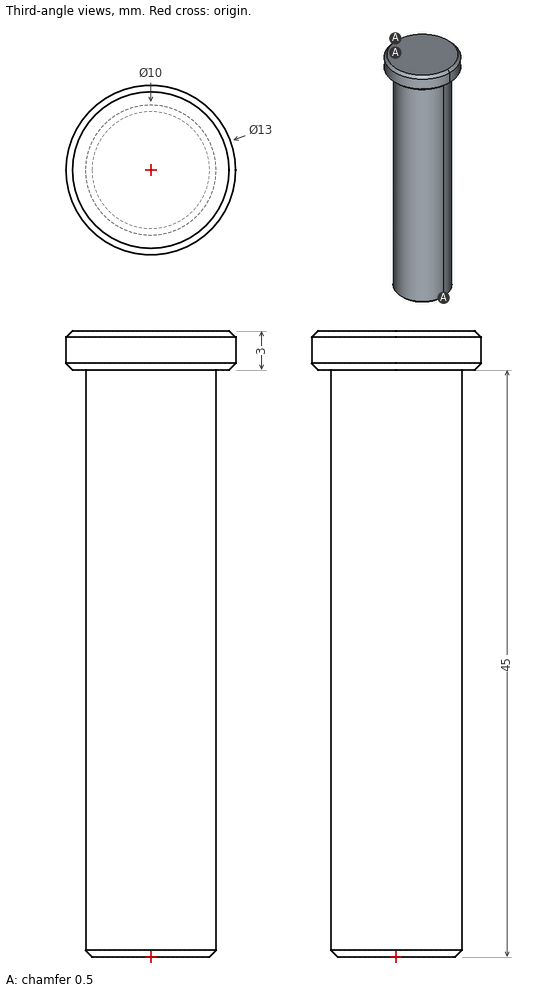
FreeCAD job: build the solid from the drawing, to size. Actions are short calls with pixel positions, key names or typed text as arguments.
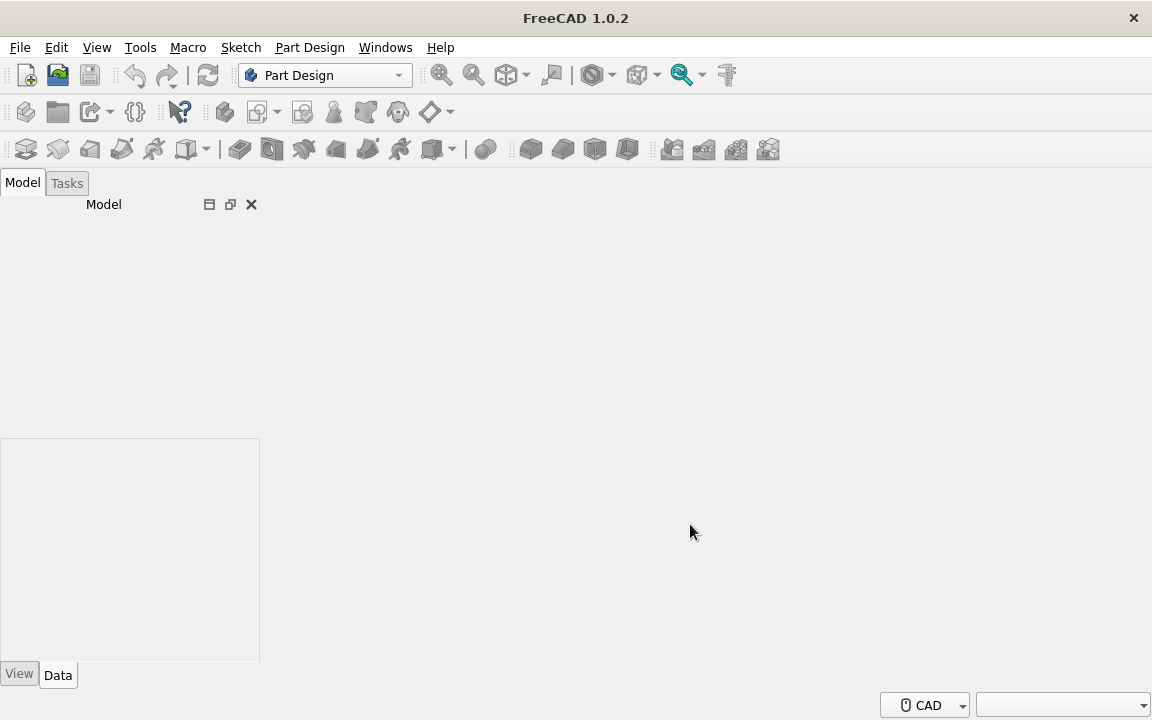
key(ctrl+n)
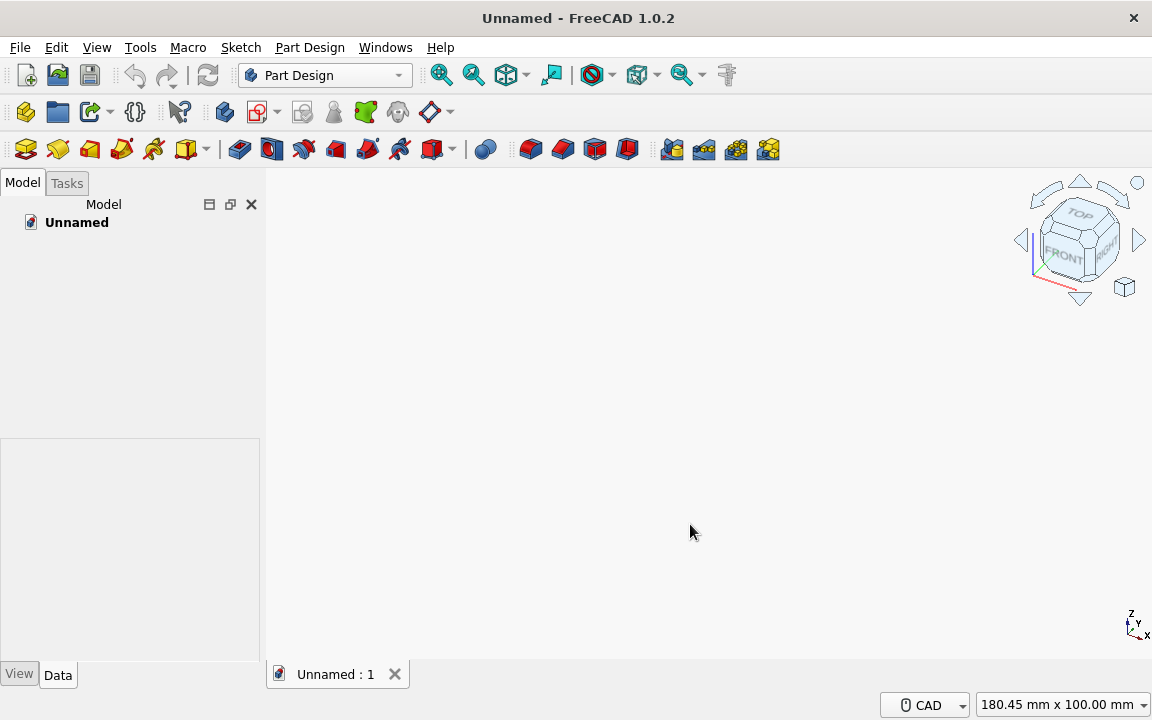
click(258, 112)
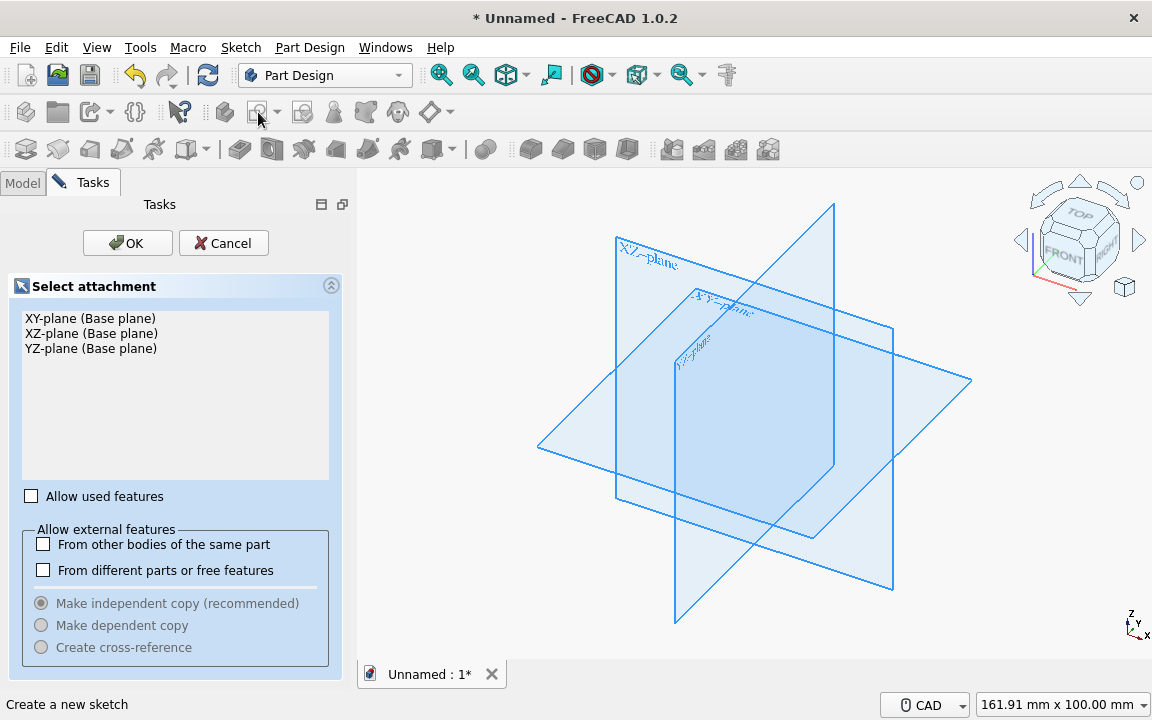
click(82, 318)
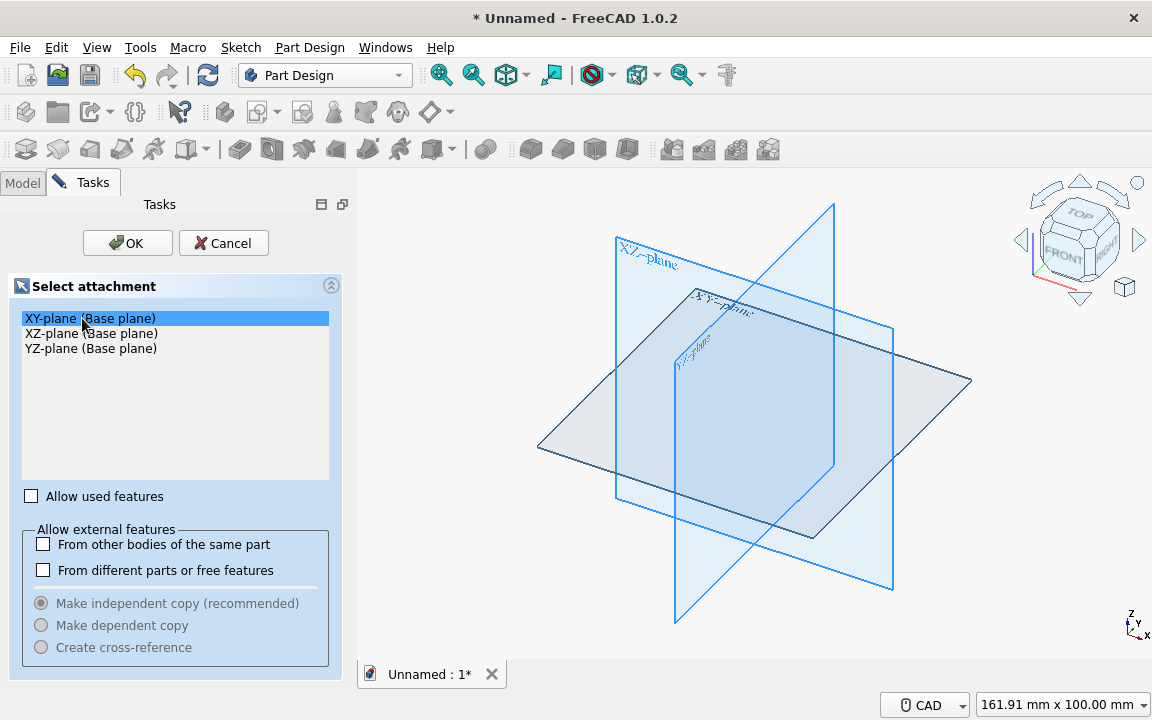
click(128, 243)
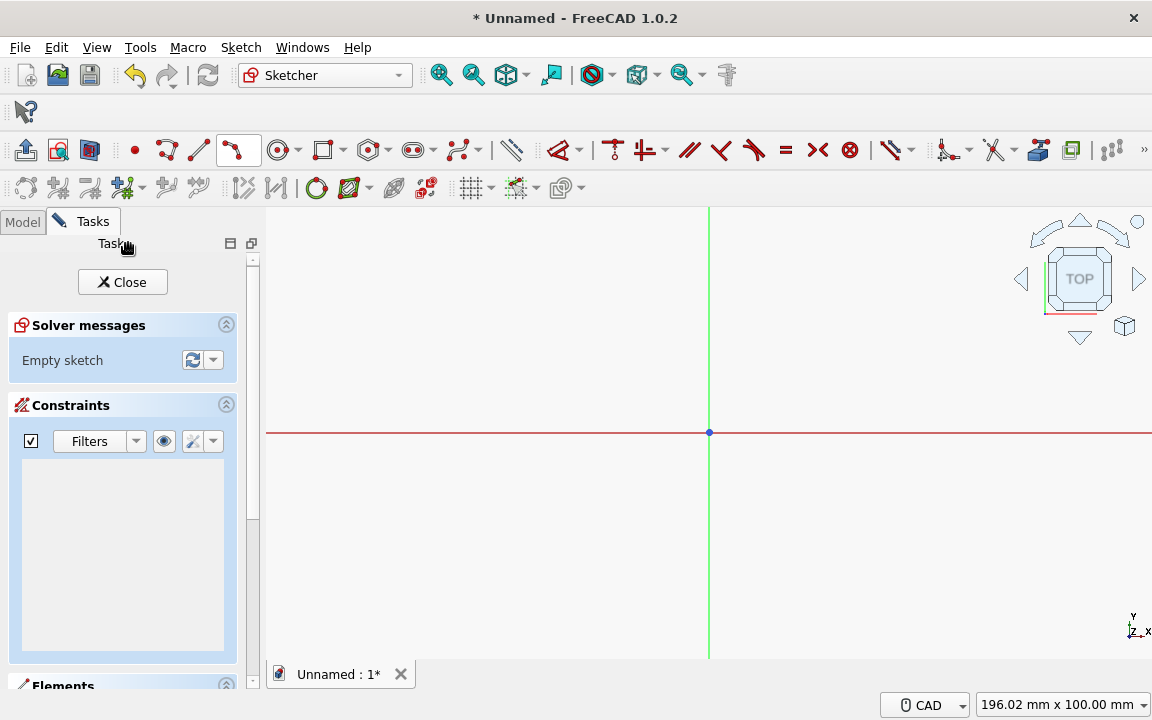
scroll(723, 433, up, 9)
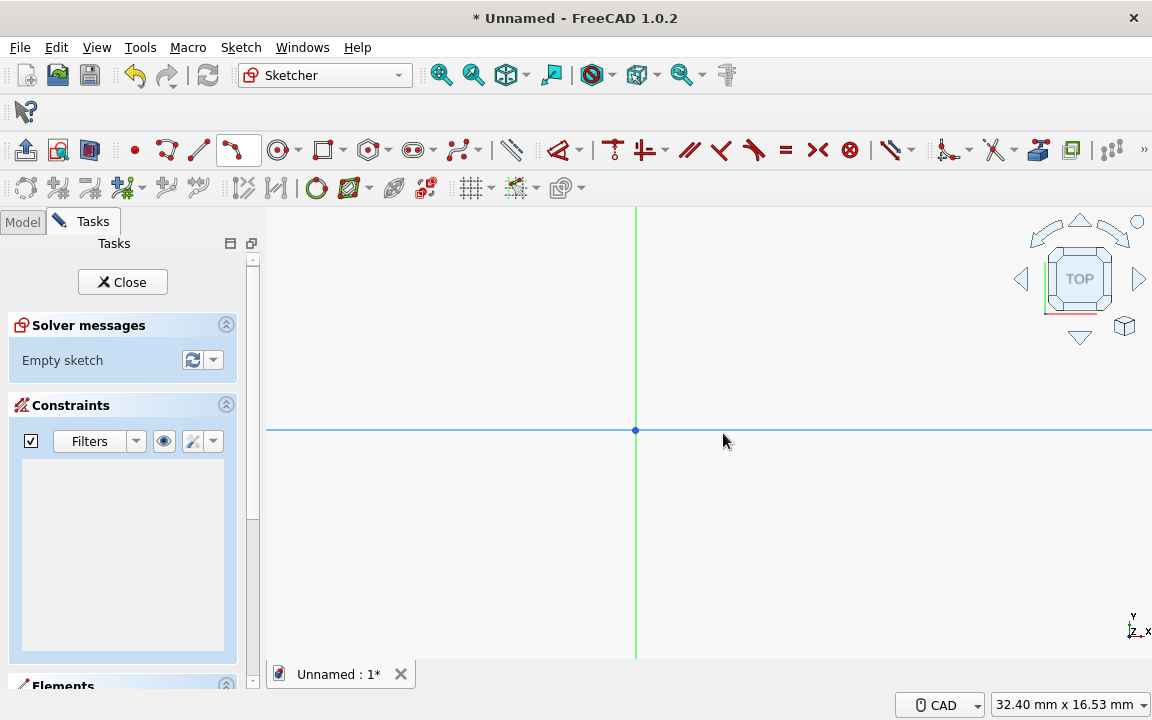
click(278, 150)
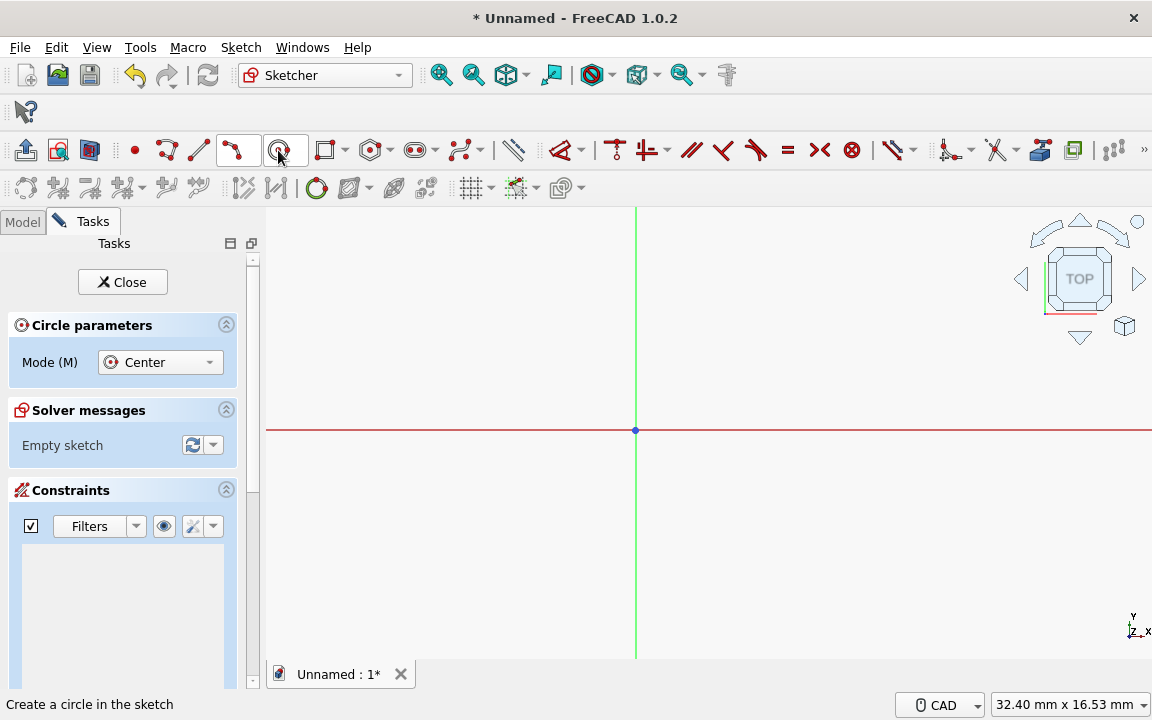
click(636, 430)
move(732, 334)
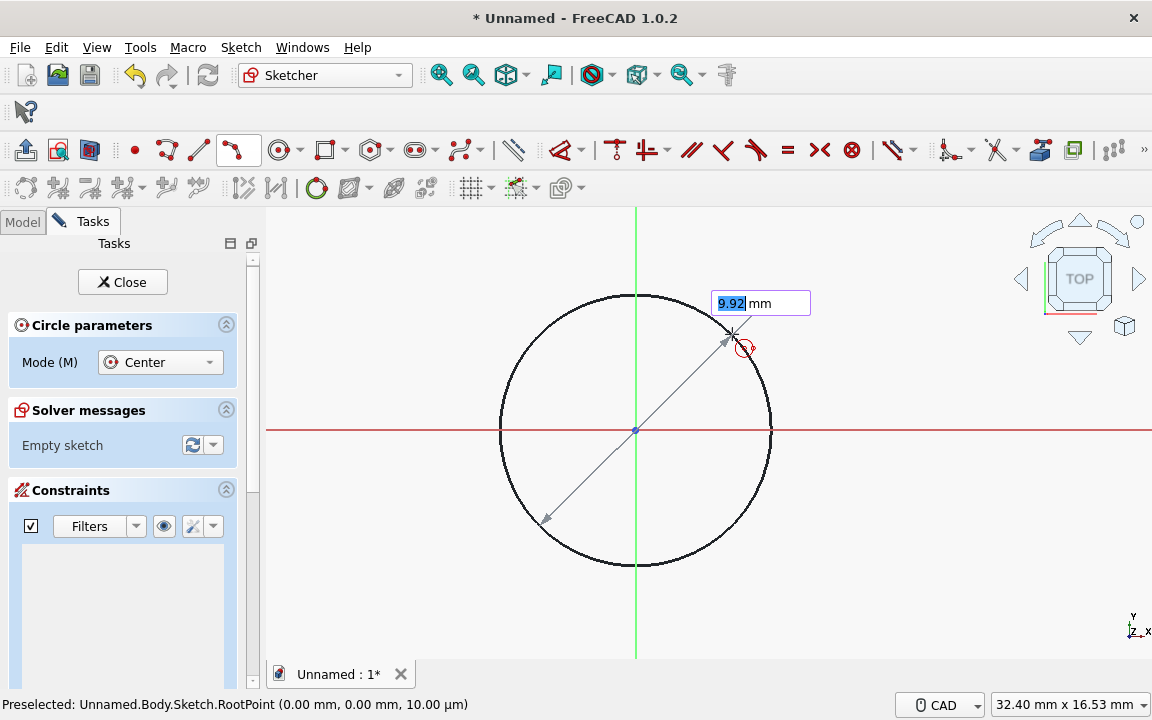
text(10)
key(Return)
key(Escape)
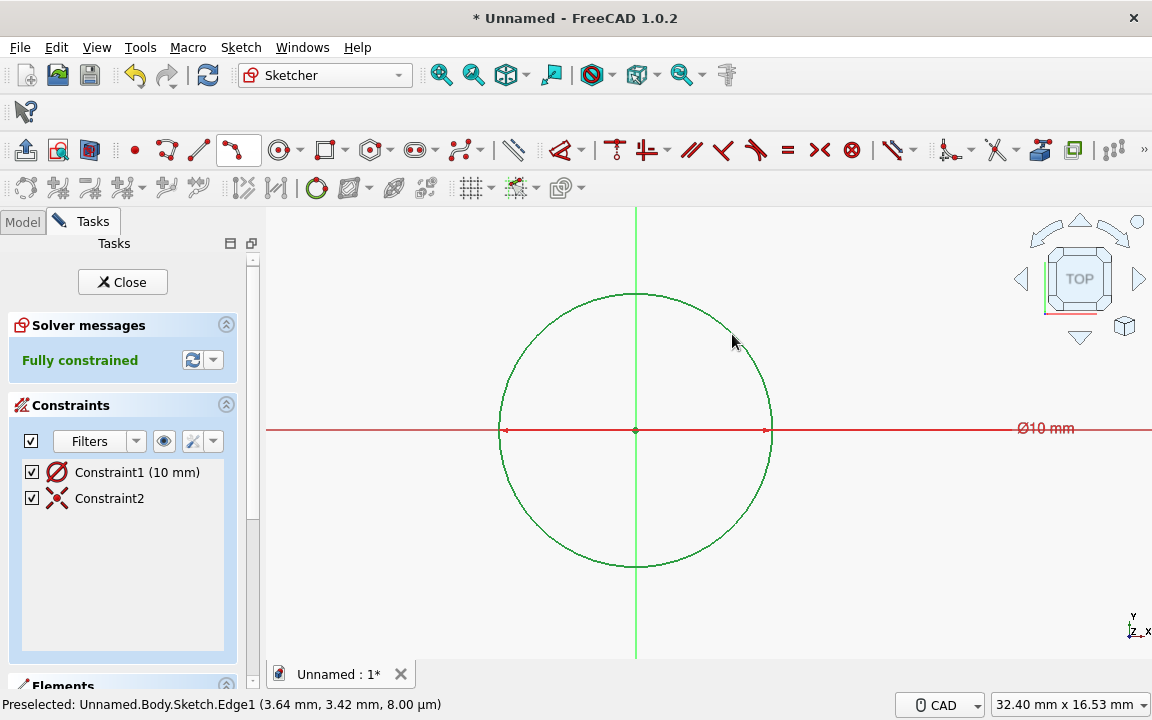
click(123, 282)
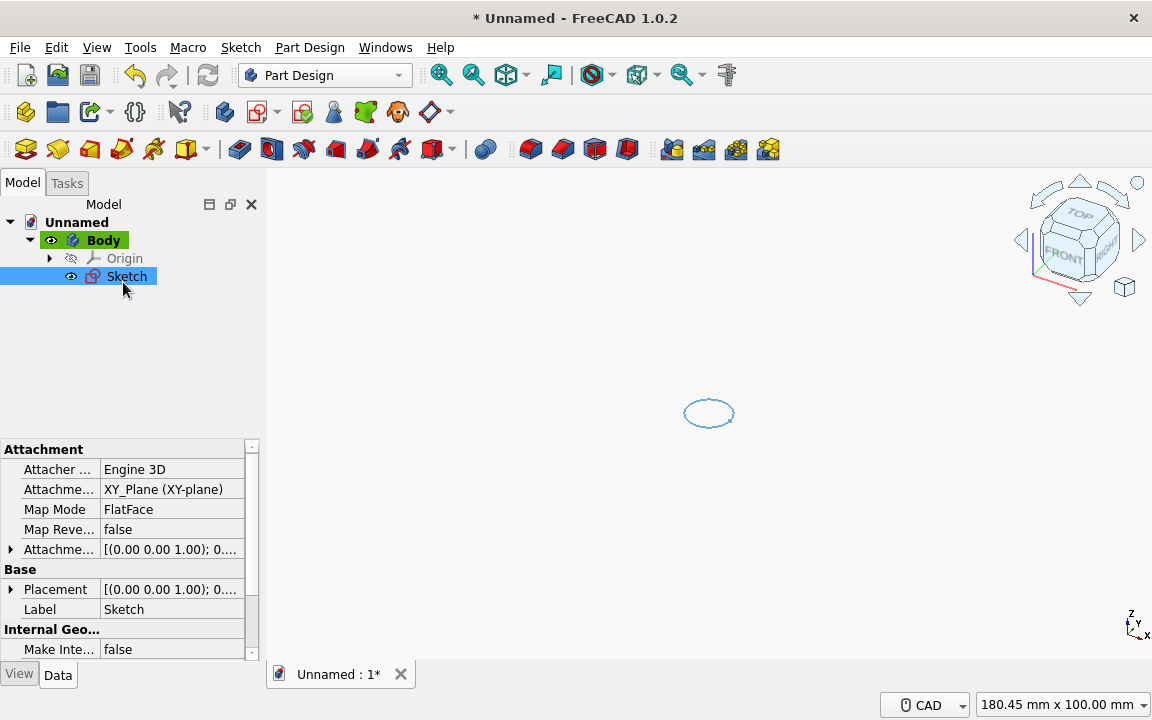
click(26, 150)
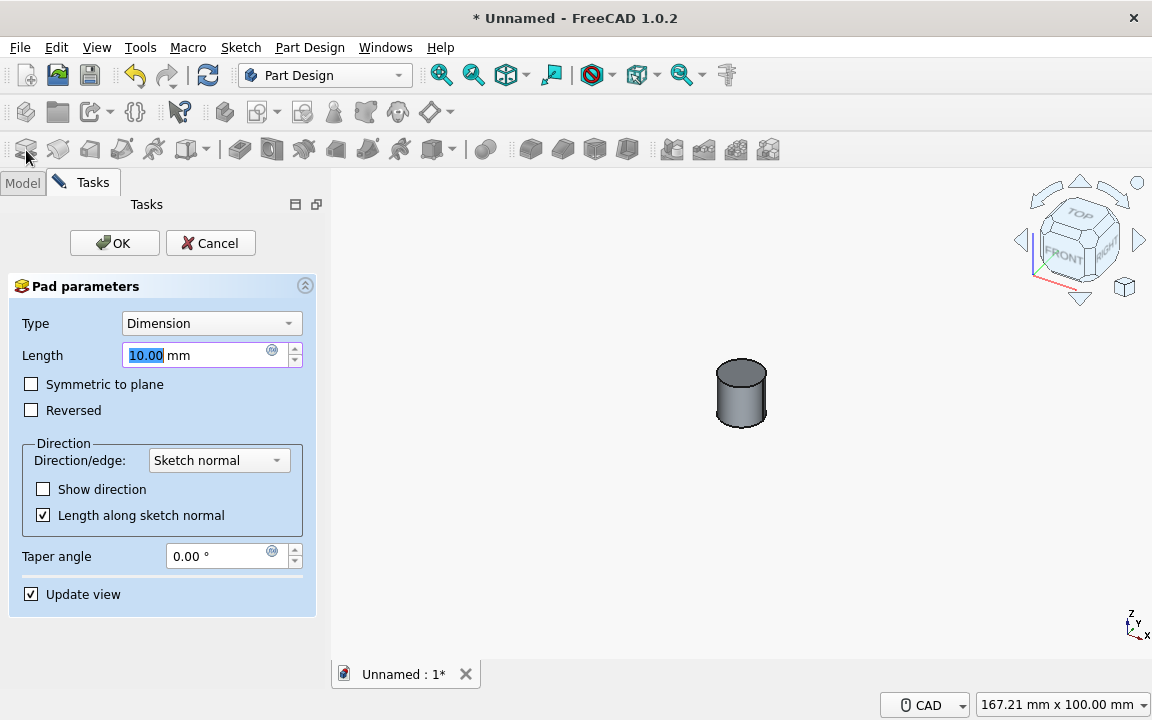
text(45)
key(Tab)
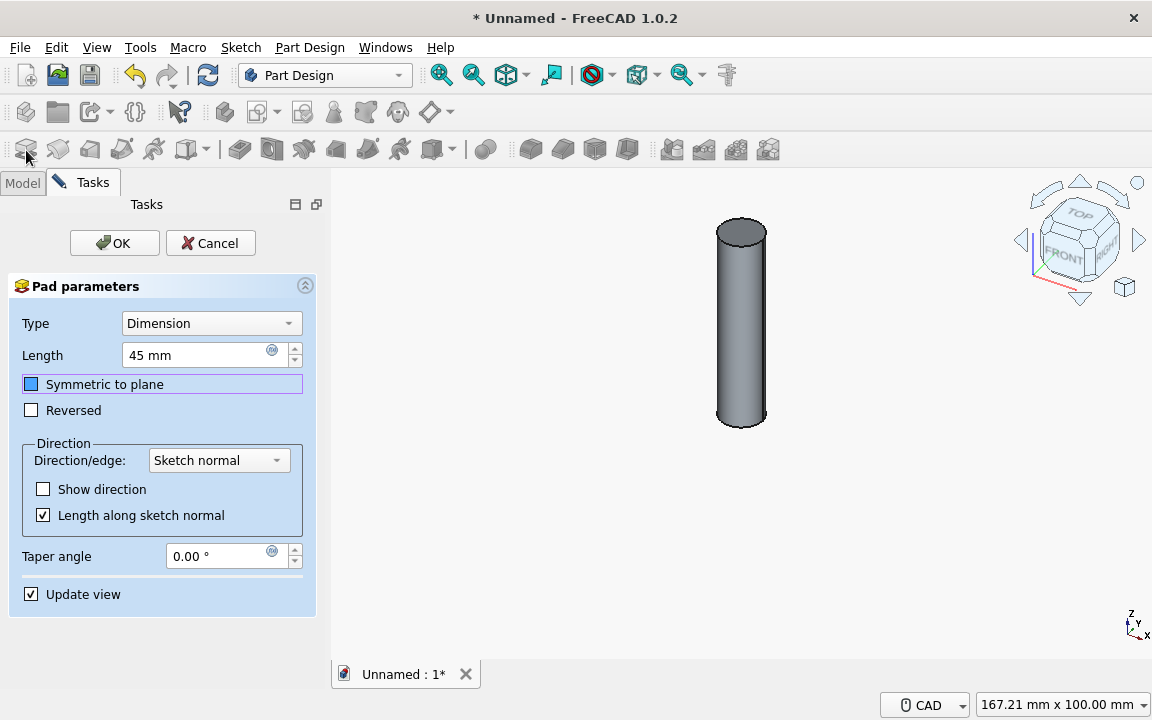
click(115, 243)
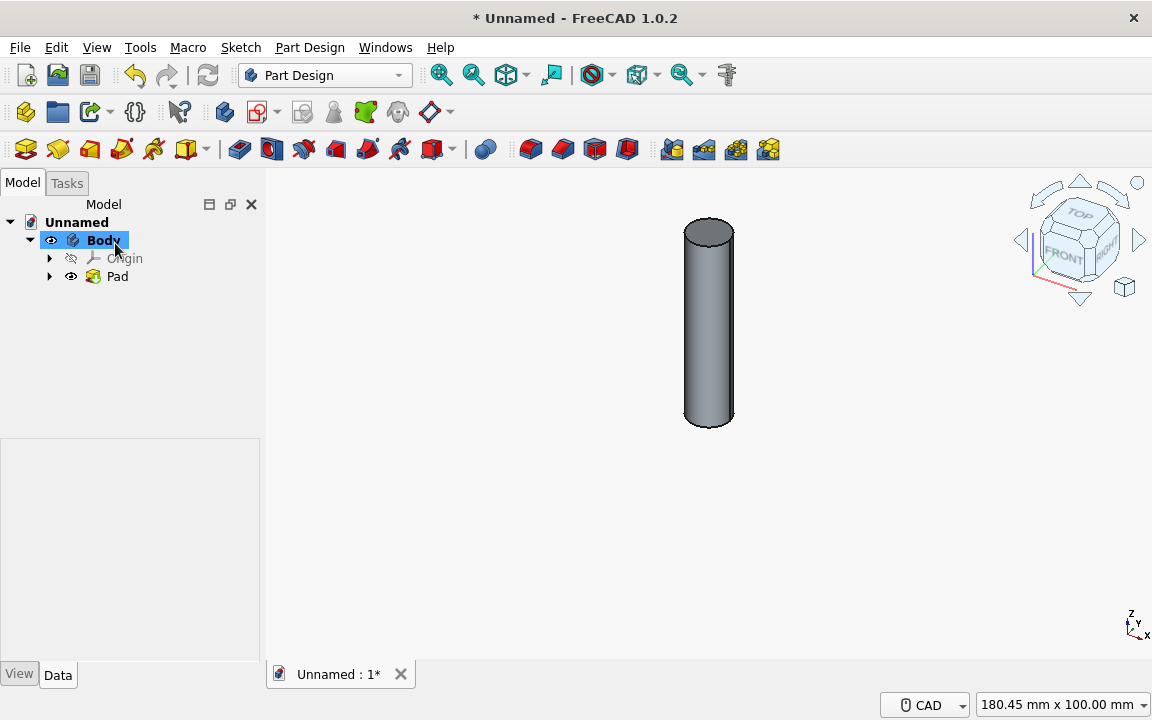
key(v)
key(f)